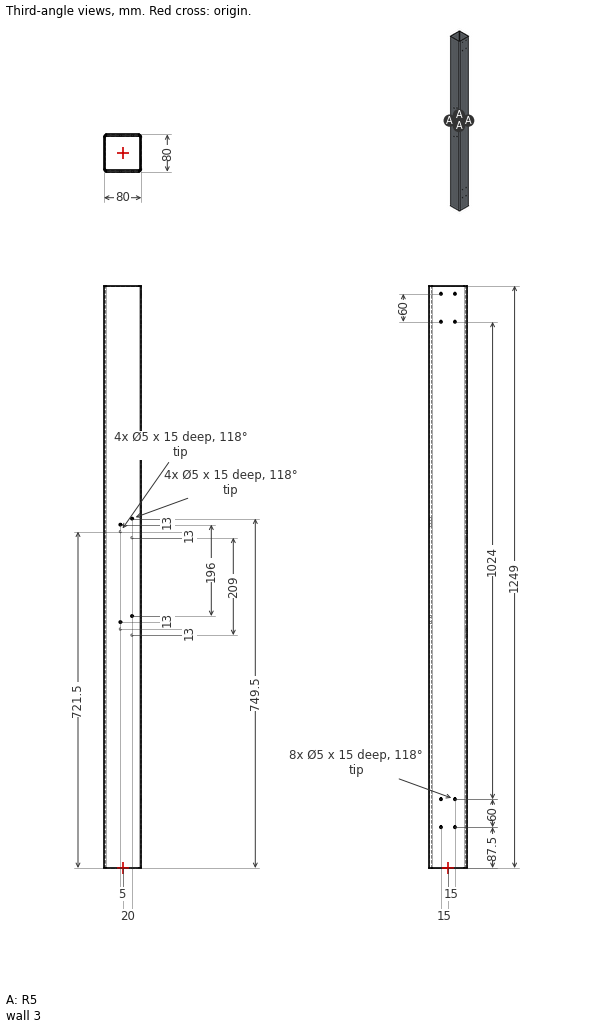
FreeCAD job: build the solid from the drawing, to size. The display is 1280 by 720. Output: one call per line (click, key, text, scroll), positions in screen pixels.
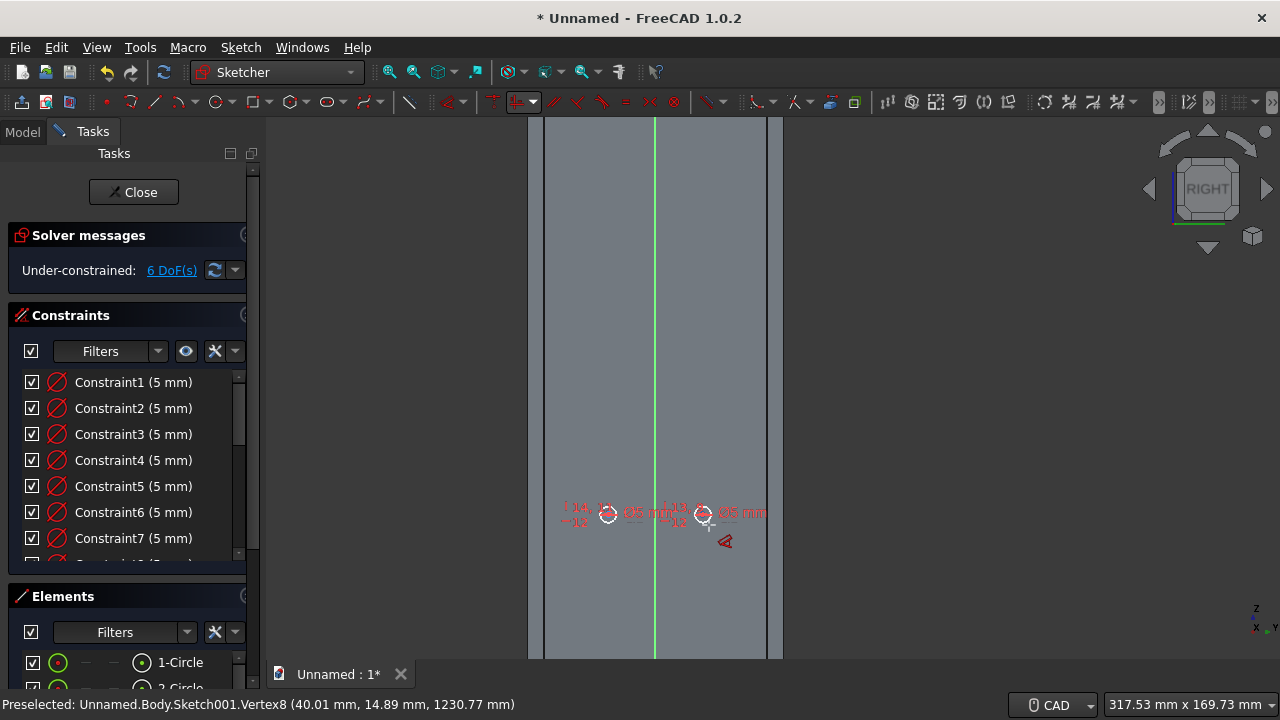
click(703, 515)
click(679, 481)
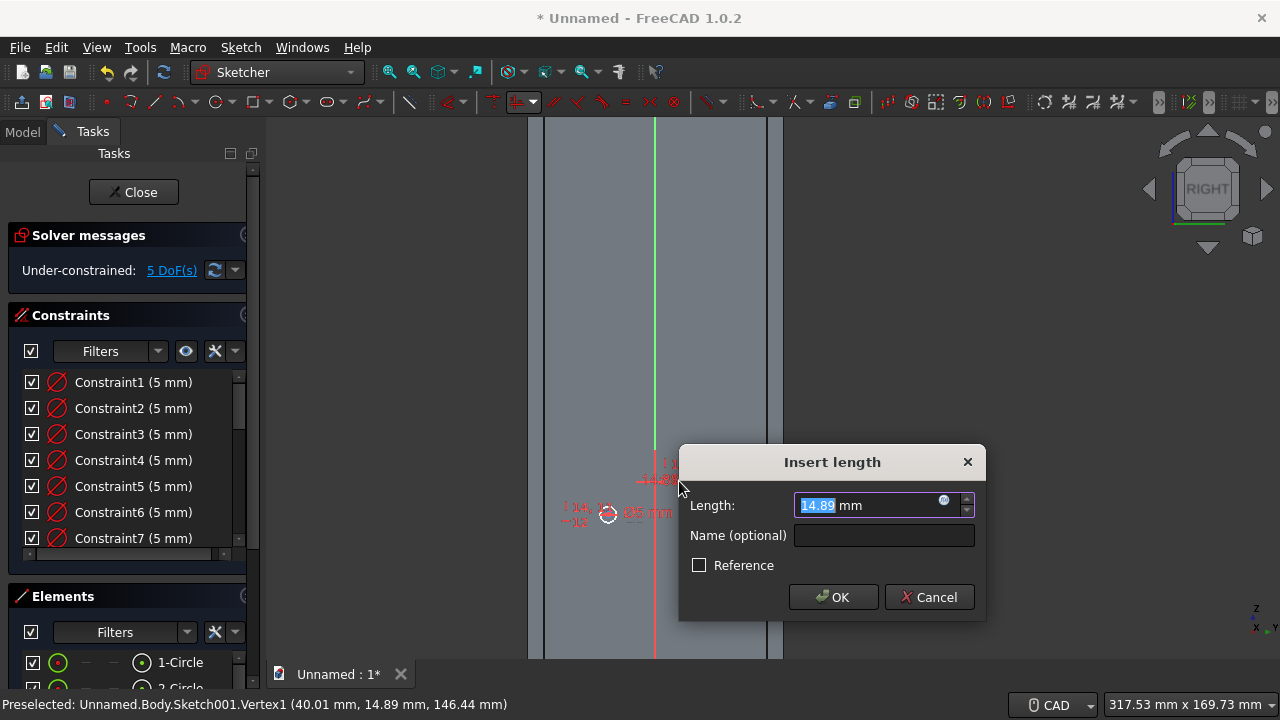
text(15)
key(Return)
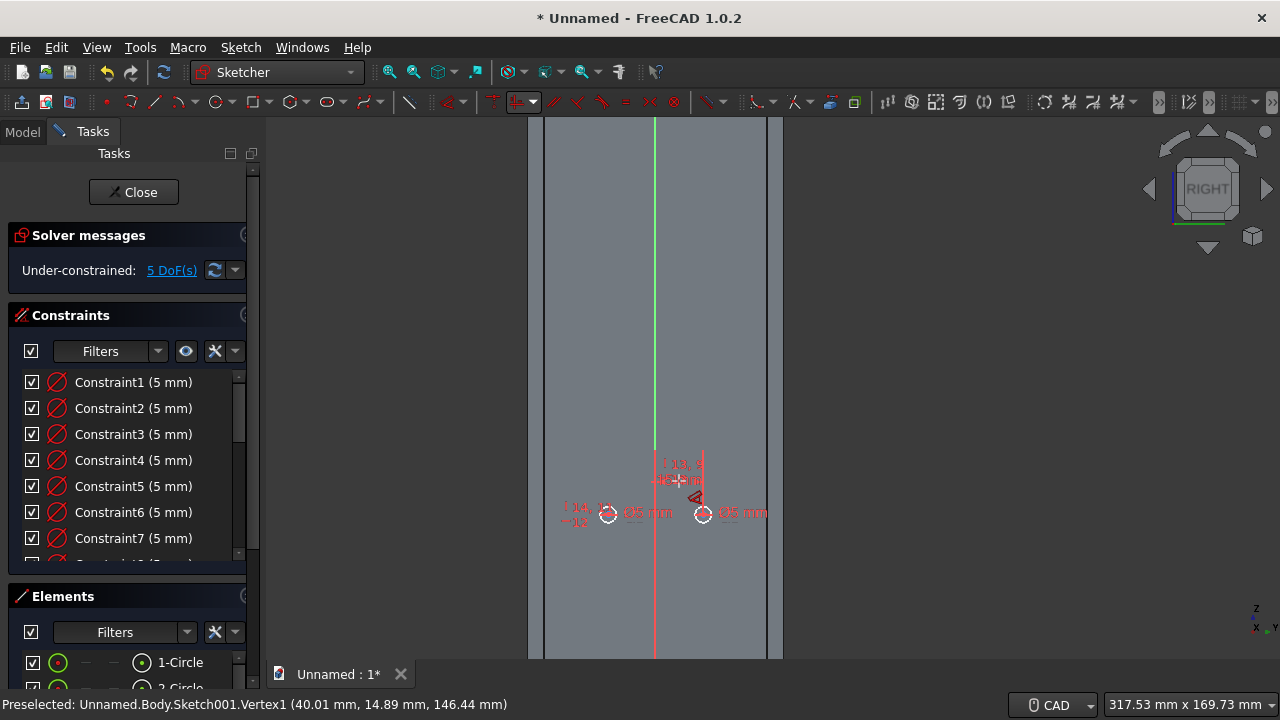
scroll(709, 525, down, 12)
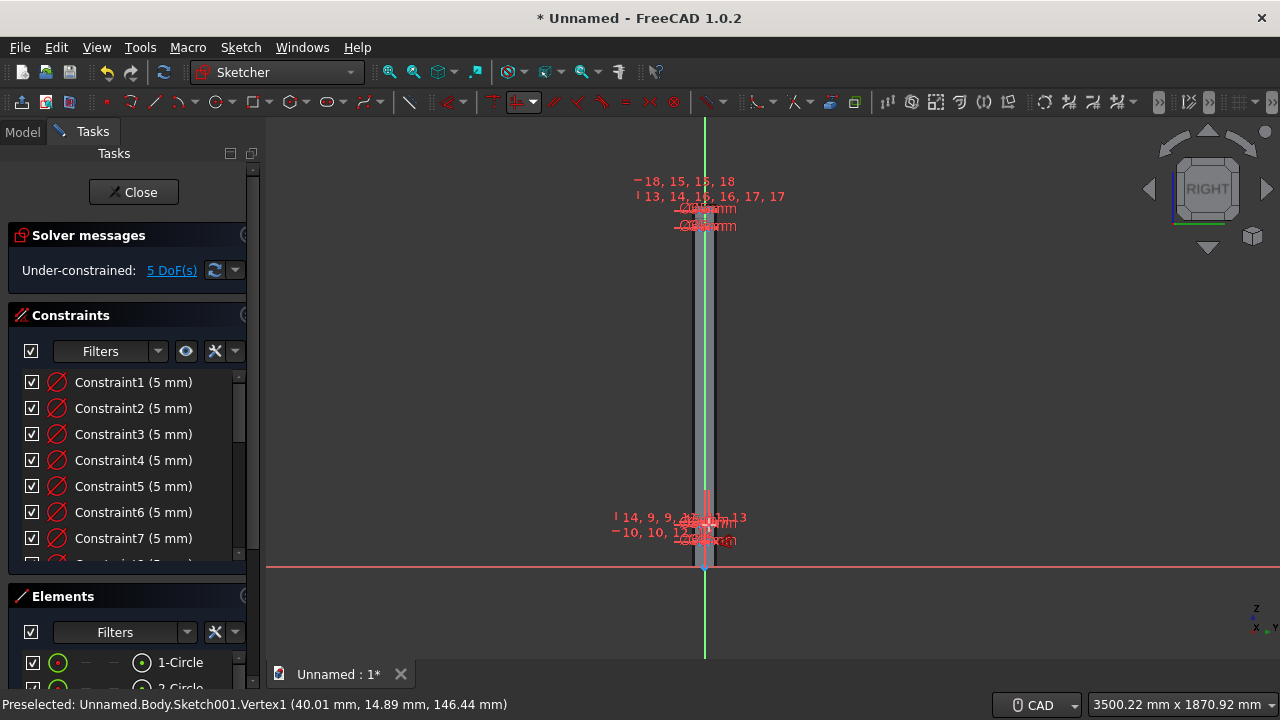
scroll(700, 542, up, 12)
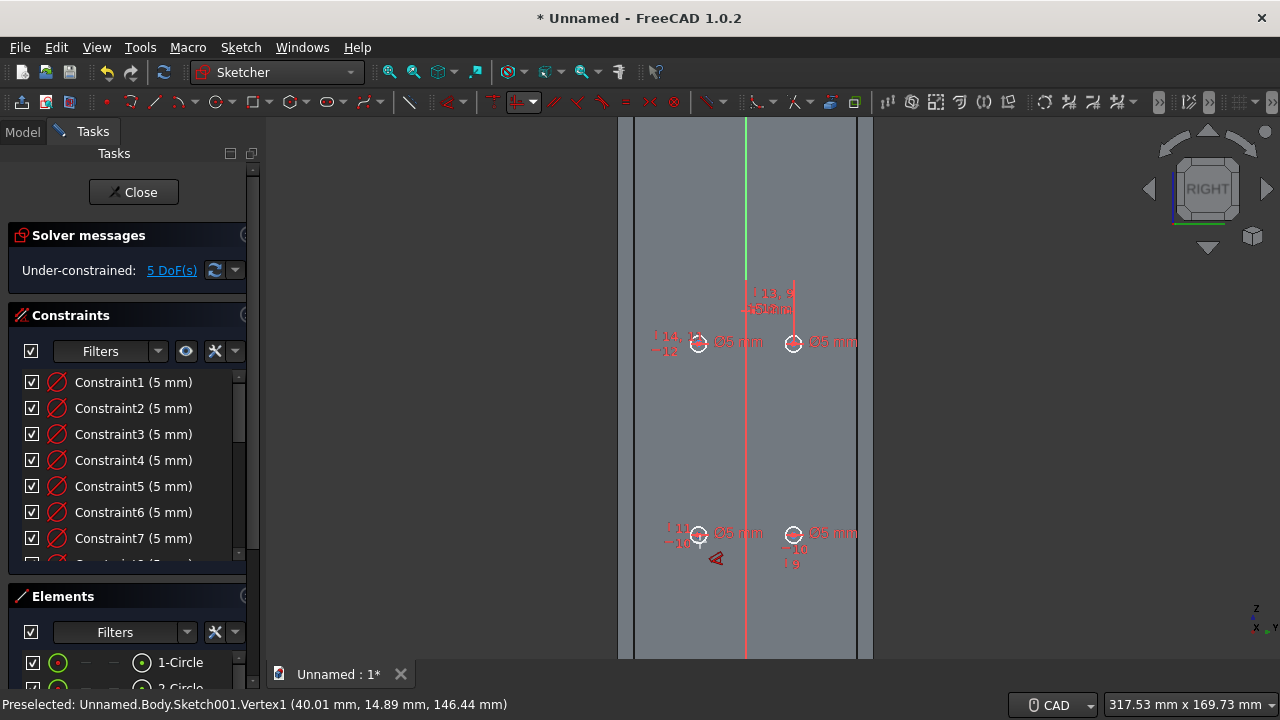
click(699, 535)
click(722, 501)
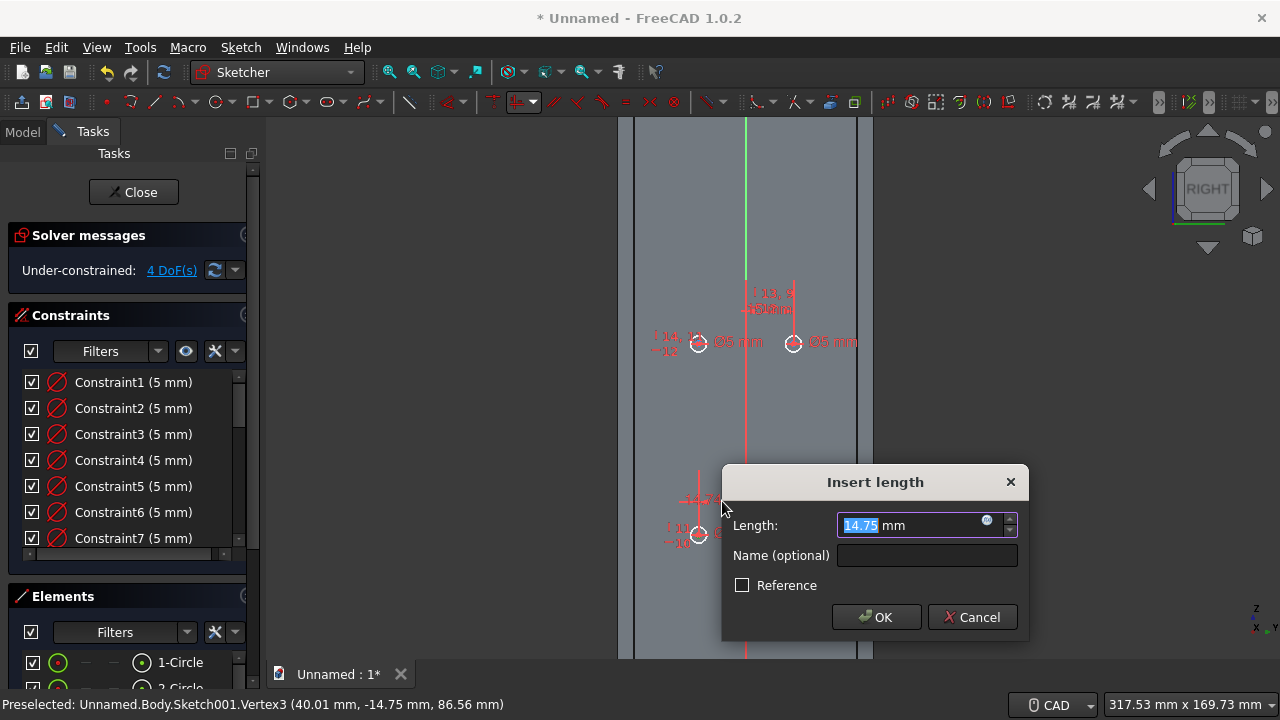
text(15)
key(Return)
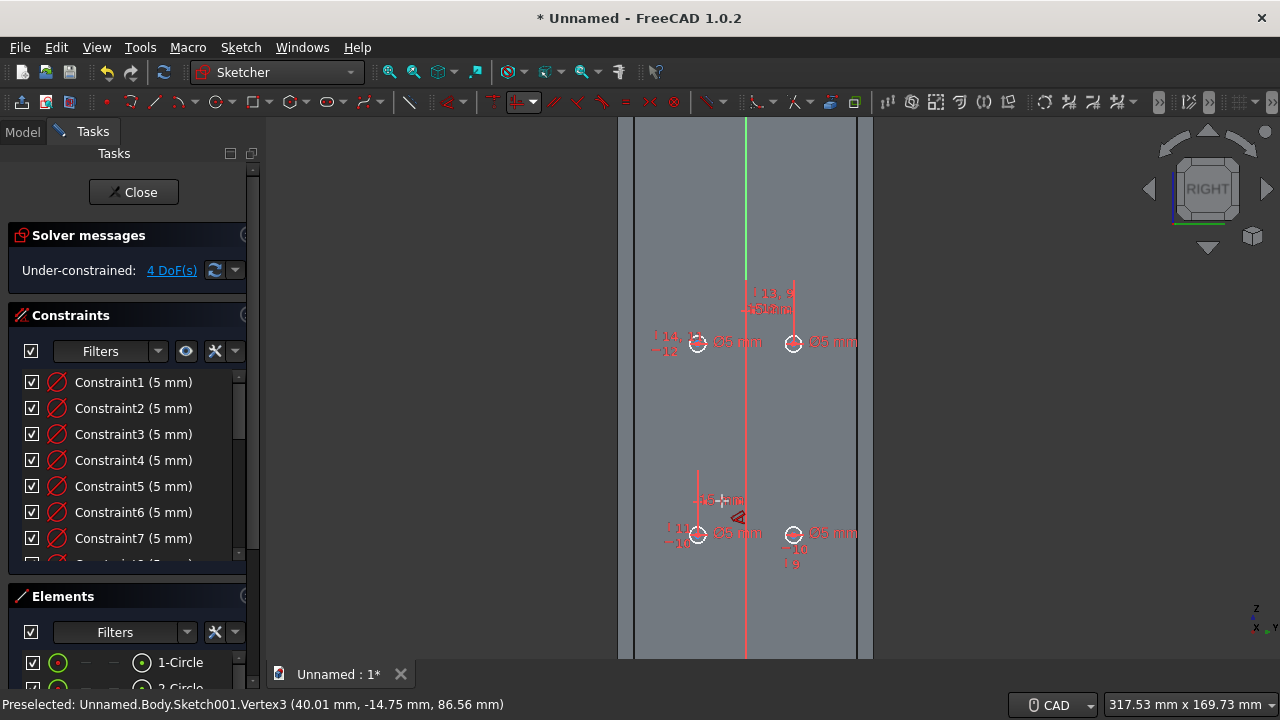
scroll(700, 542, down, 12)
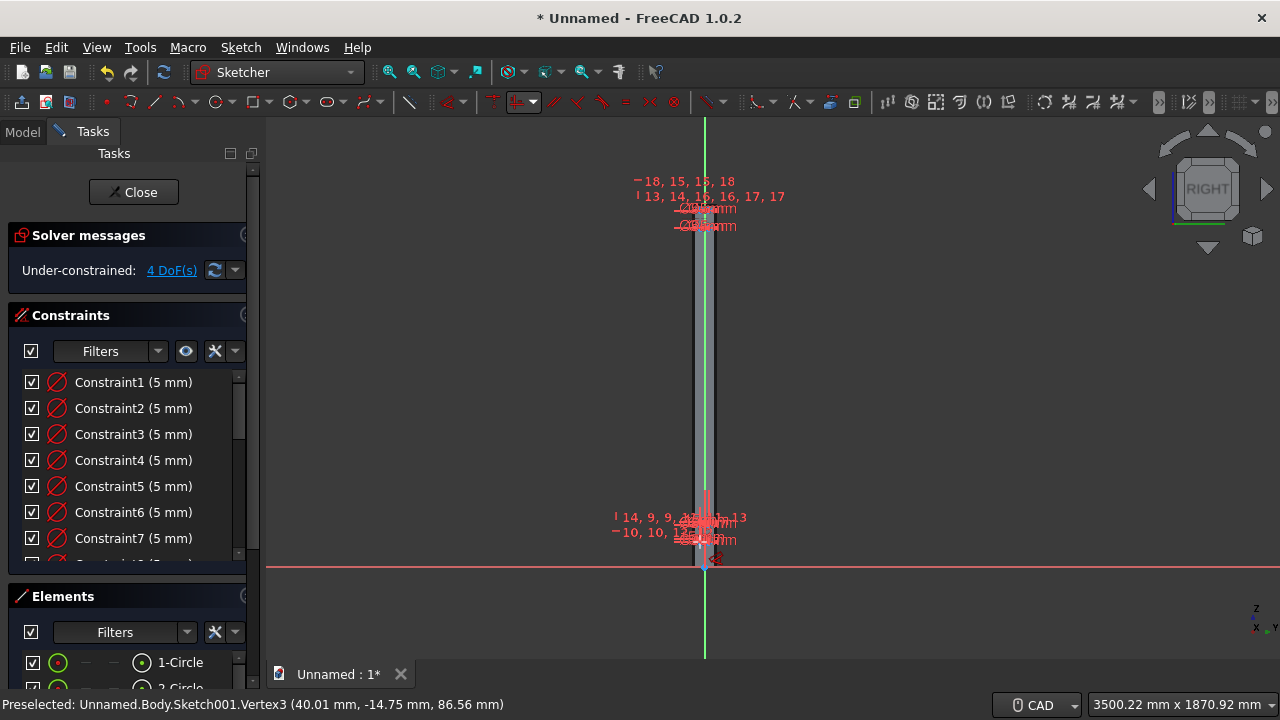
scroll(709, 525, up, 5)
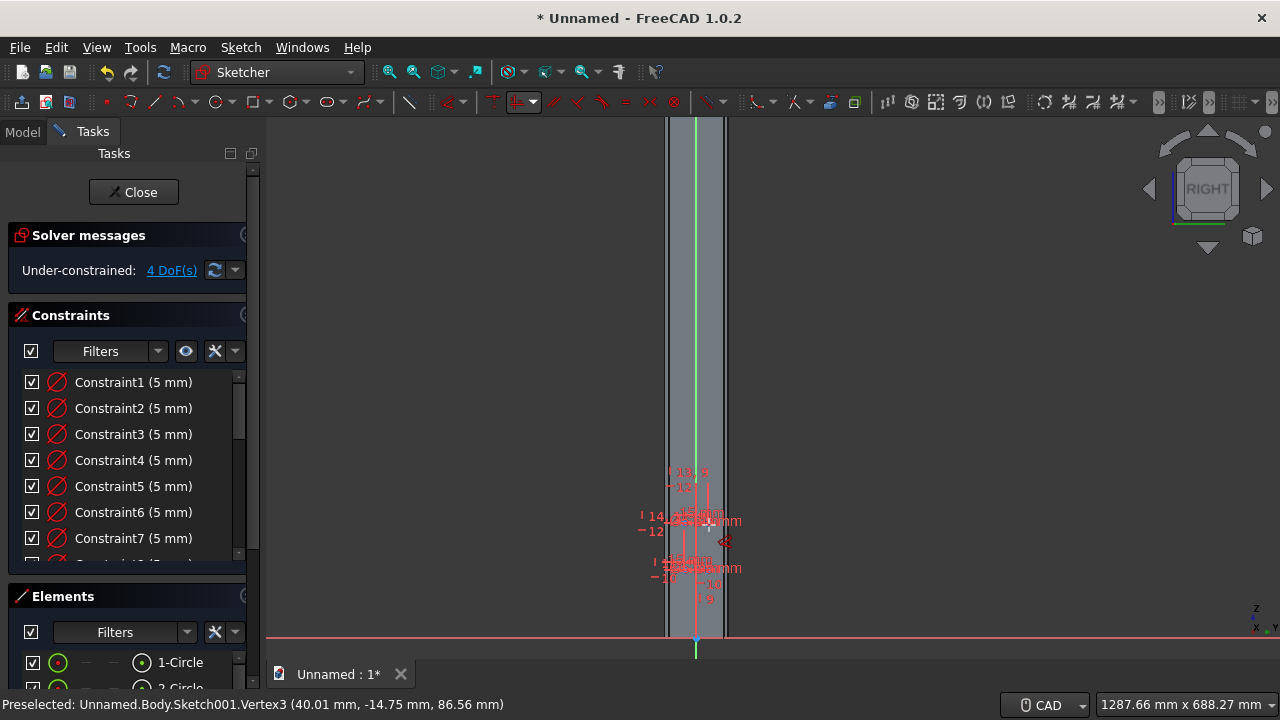
click(708, 523)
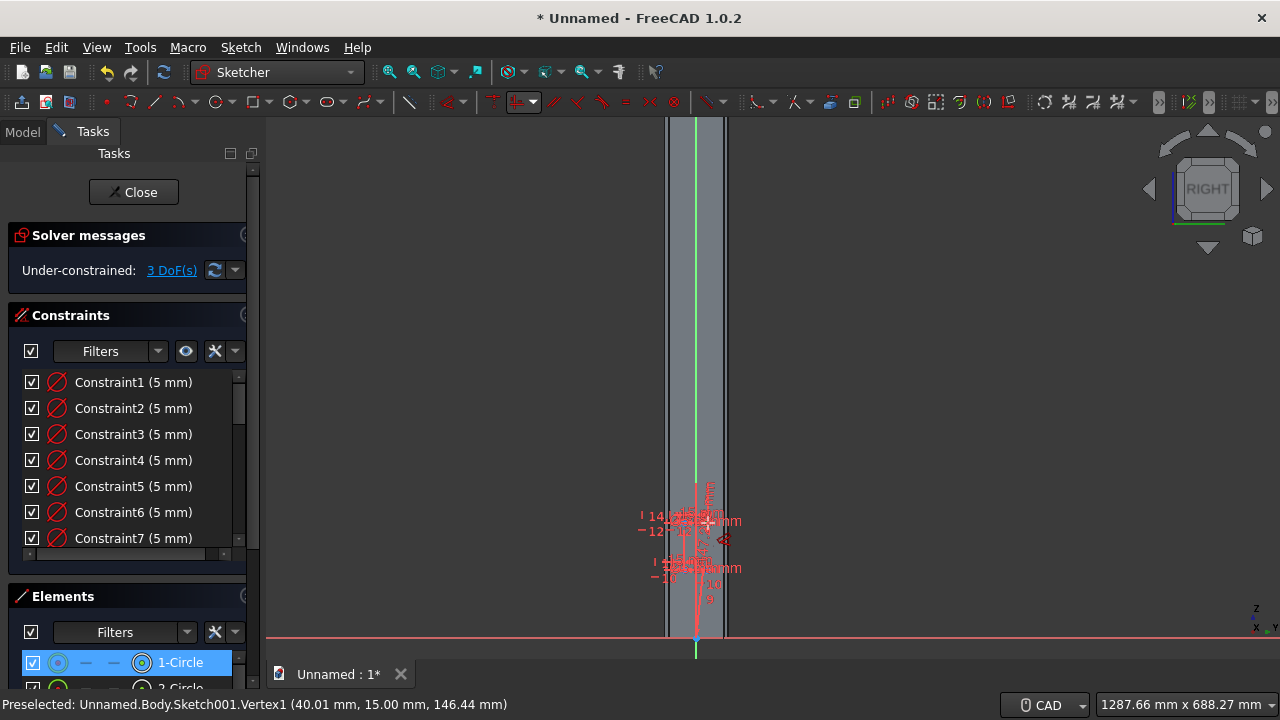
click(708, 570)
click(742, 536)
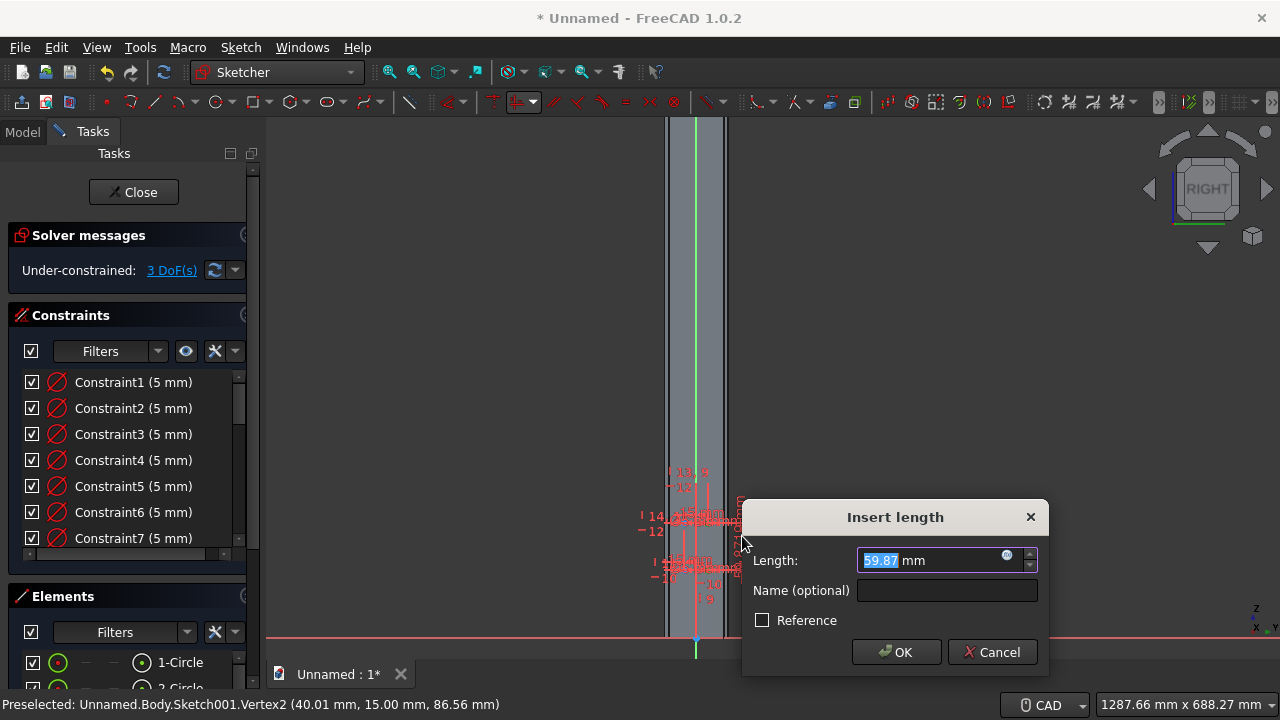
text(60)
key(Return)